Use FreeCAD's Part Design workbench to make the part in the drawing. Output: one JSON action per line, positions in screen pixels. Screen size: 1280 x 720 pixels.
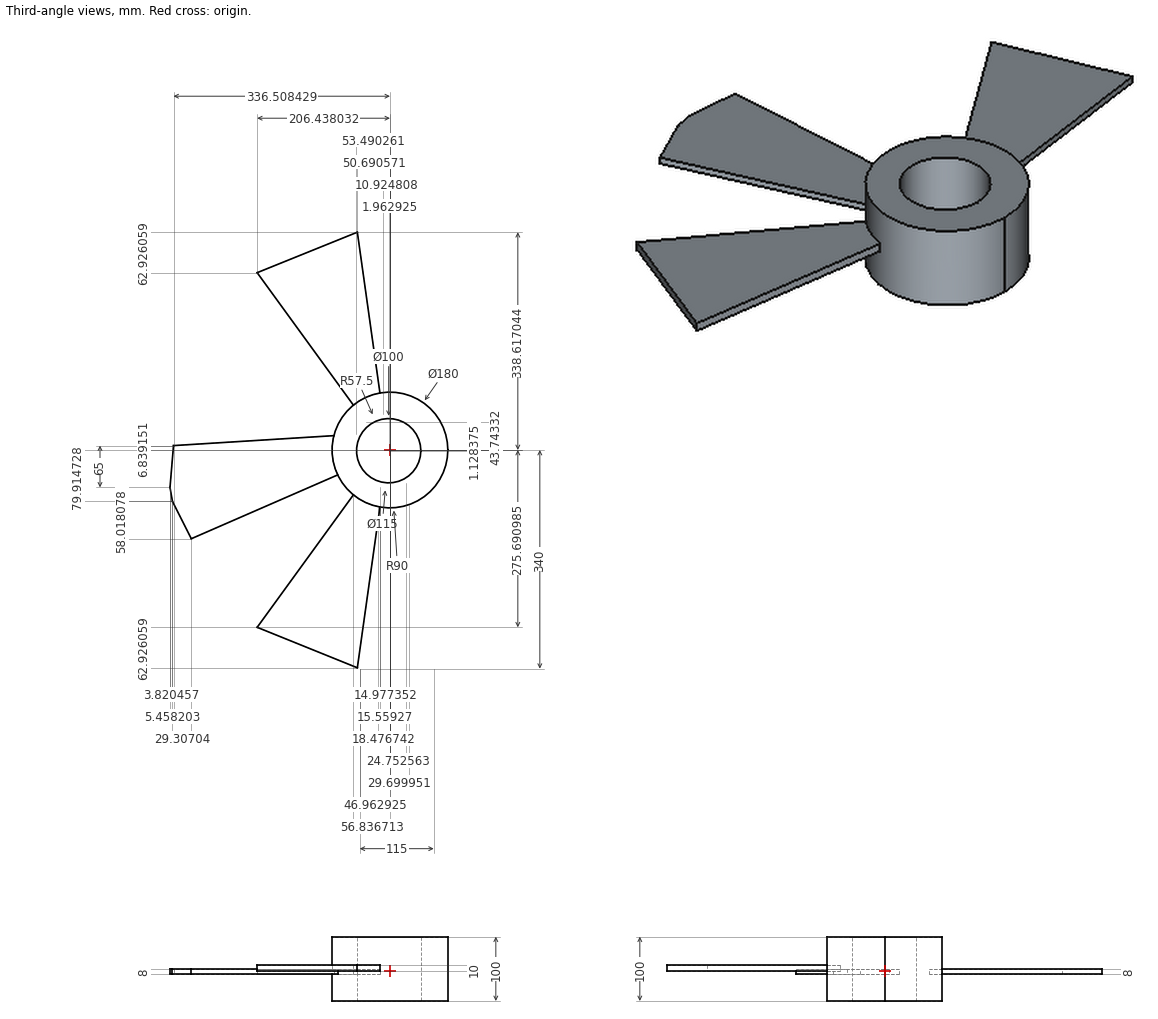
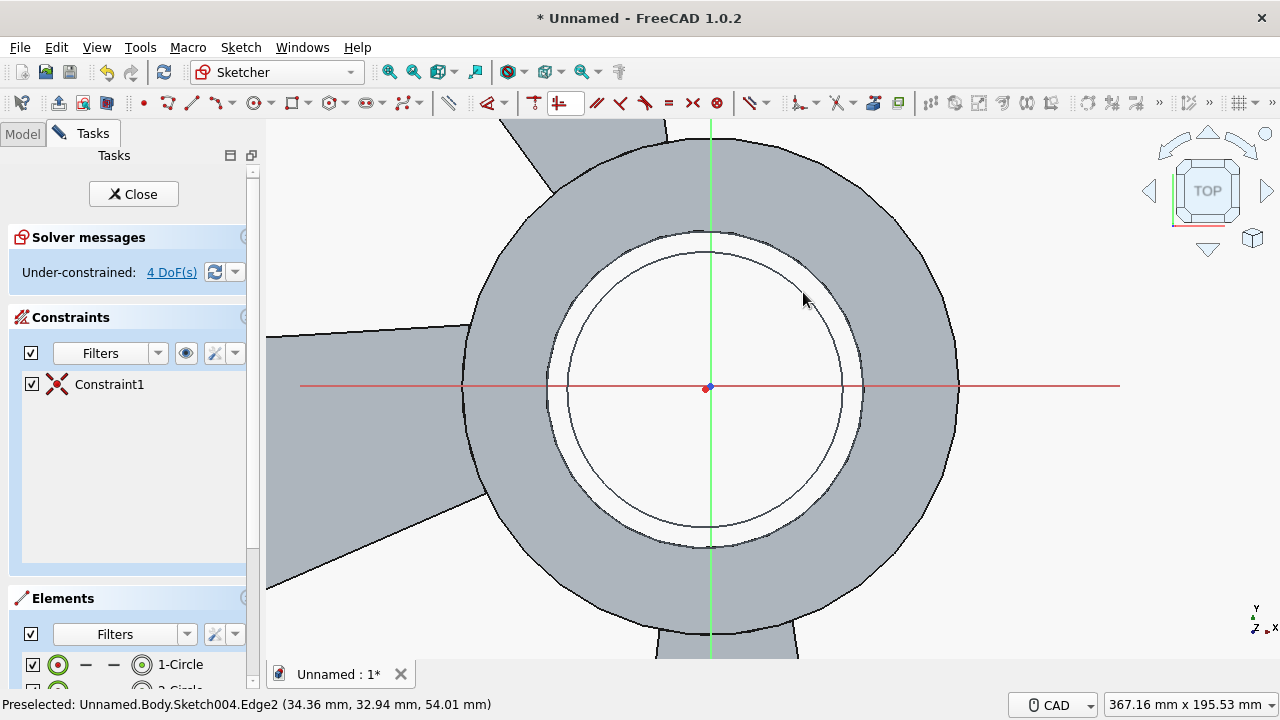
{"action": "left_click", "coordinate": [488, 104]}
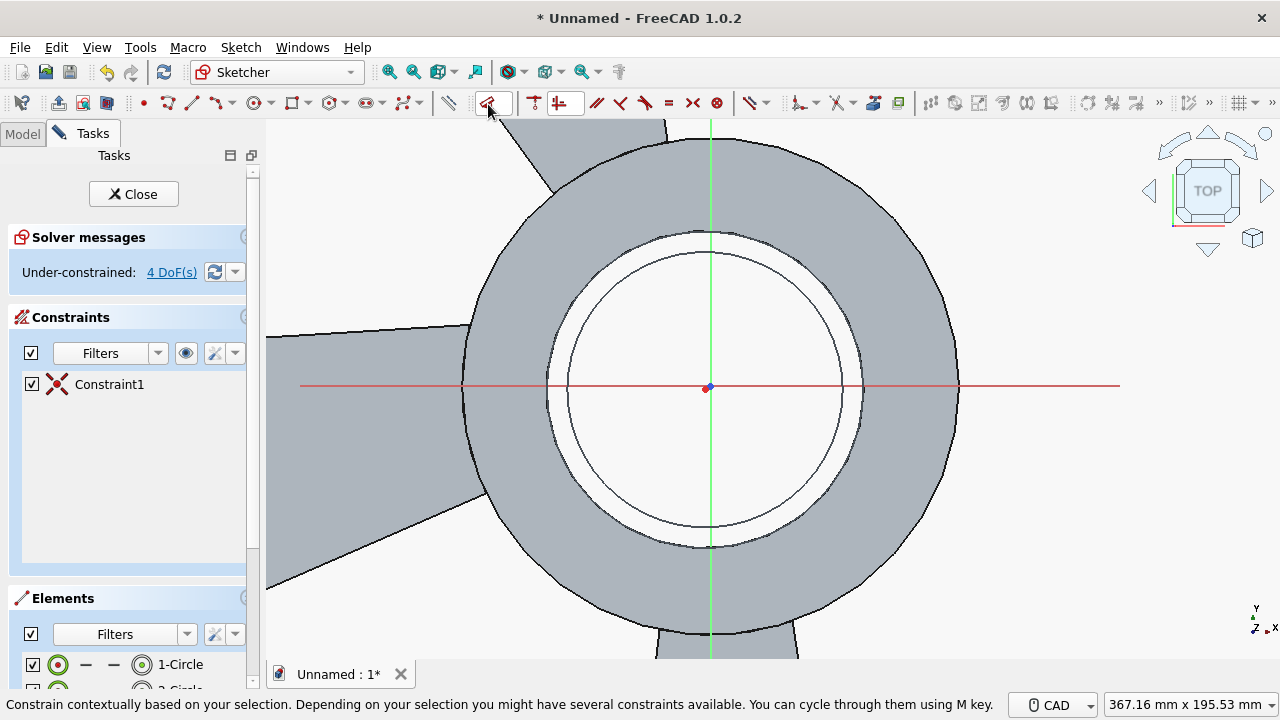
{"action": "left_click", "coordinate": [817, 278]}
{"action": "left_click", "coordinate": [840, 255]}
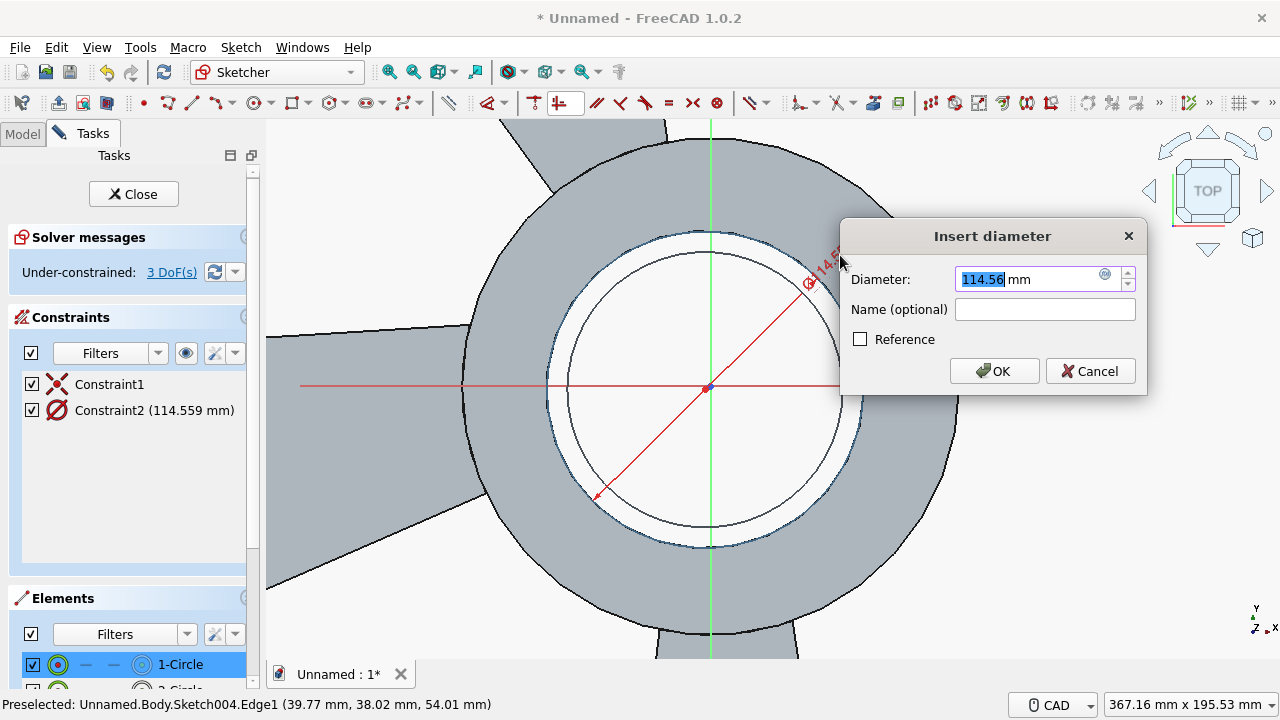
{"action": "type", "text": "115"}
{"action": "key", "text": "Return"}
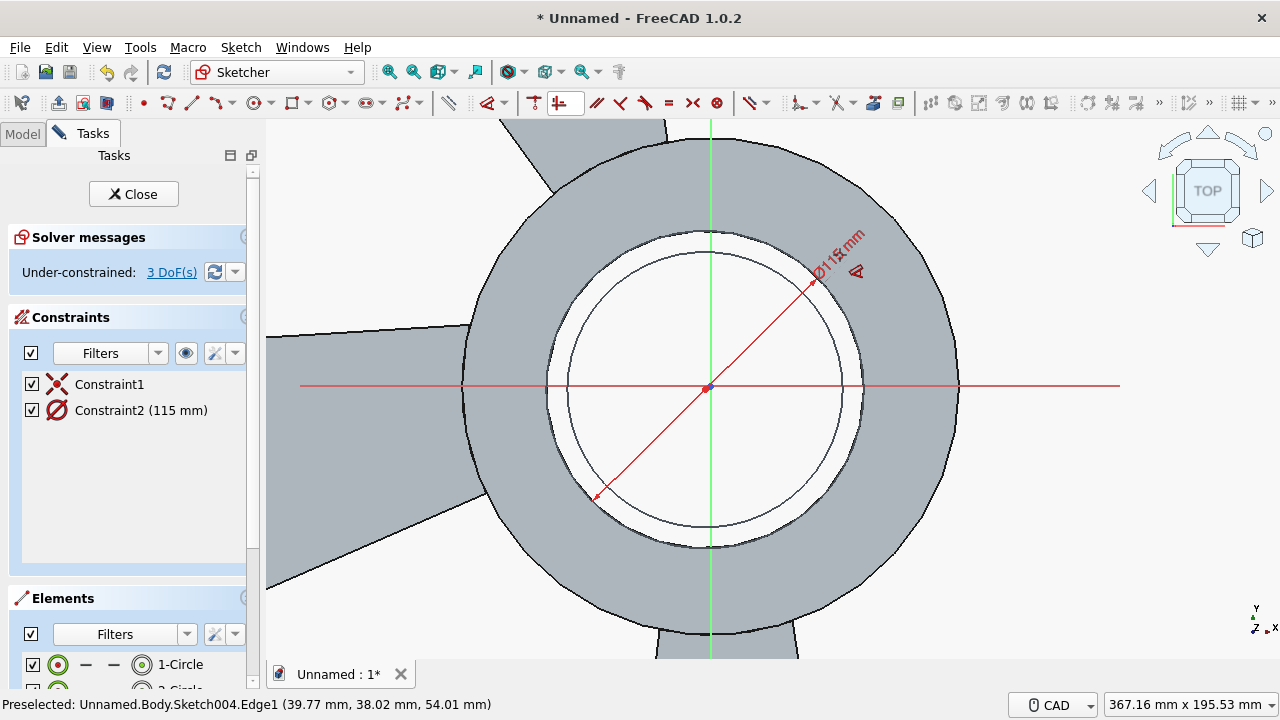
{"action": "left_click", "coordinate": [802, 292]}
{"action": "left_click", "coordinate": [890, 335]}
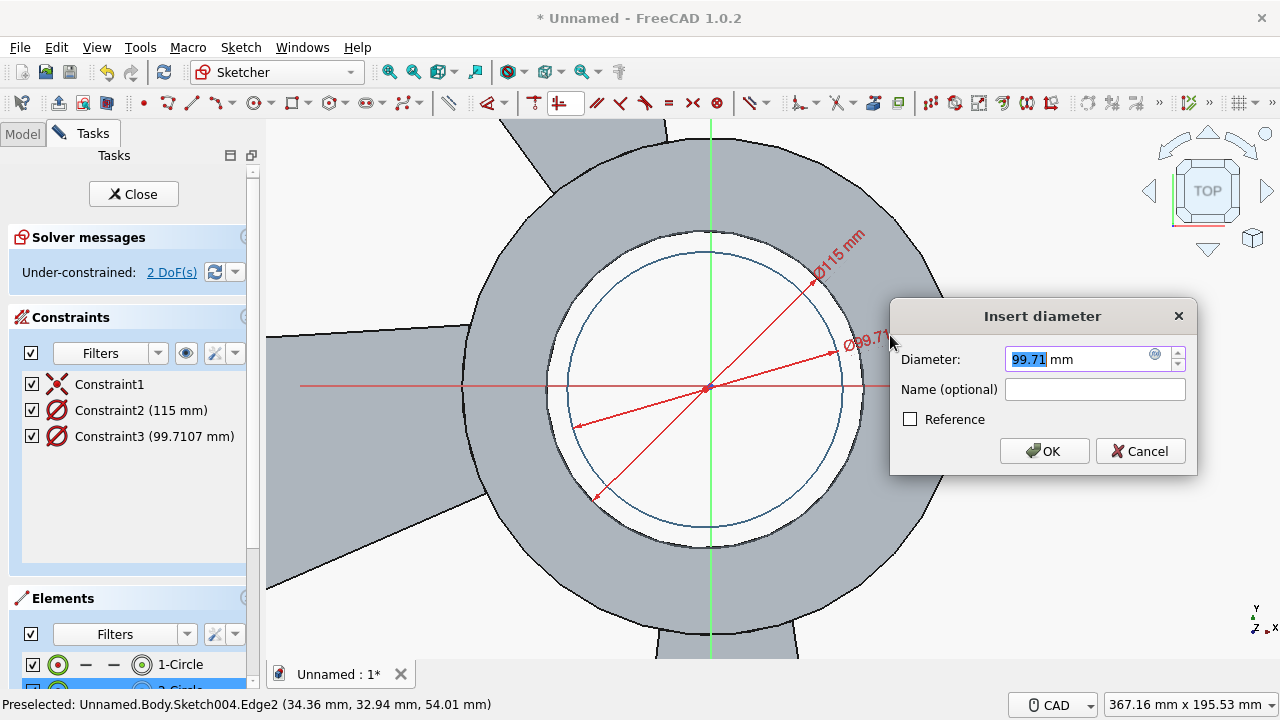
{"action": "type", "text": "100"}
{"action": "key", "text": "Return"}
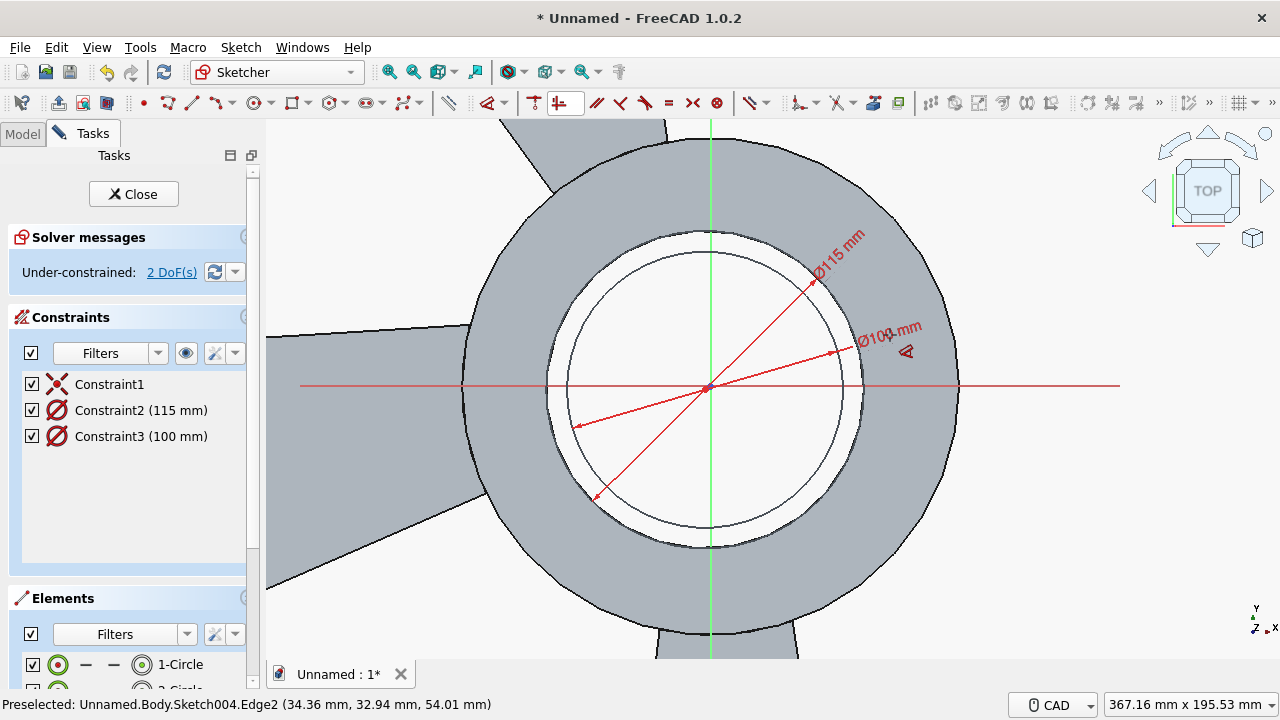
{"action": "scroll", "coordinate": [705, 390], "scroll_direction": "up", "scroll_amount": 10}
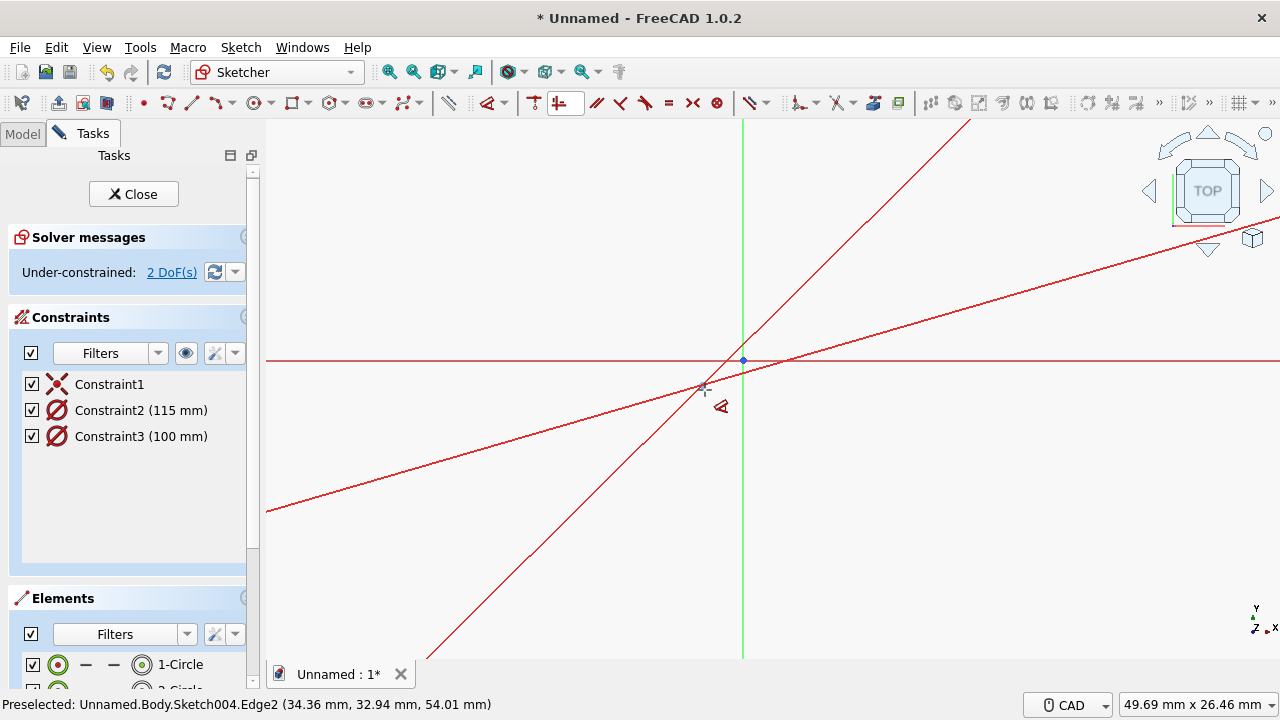
{"action": "left_click", "coordinate": [703, 385]}
{"action": "left_click", "coordinate": [723, 327]}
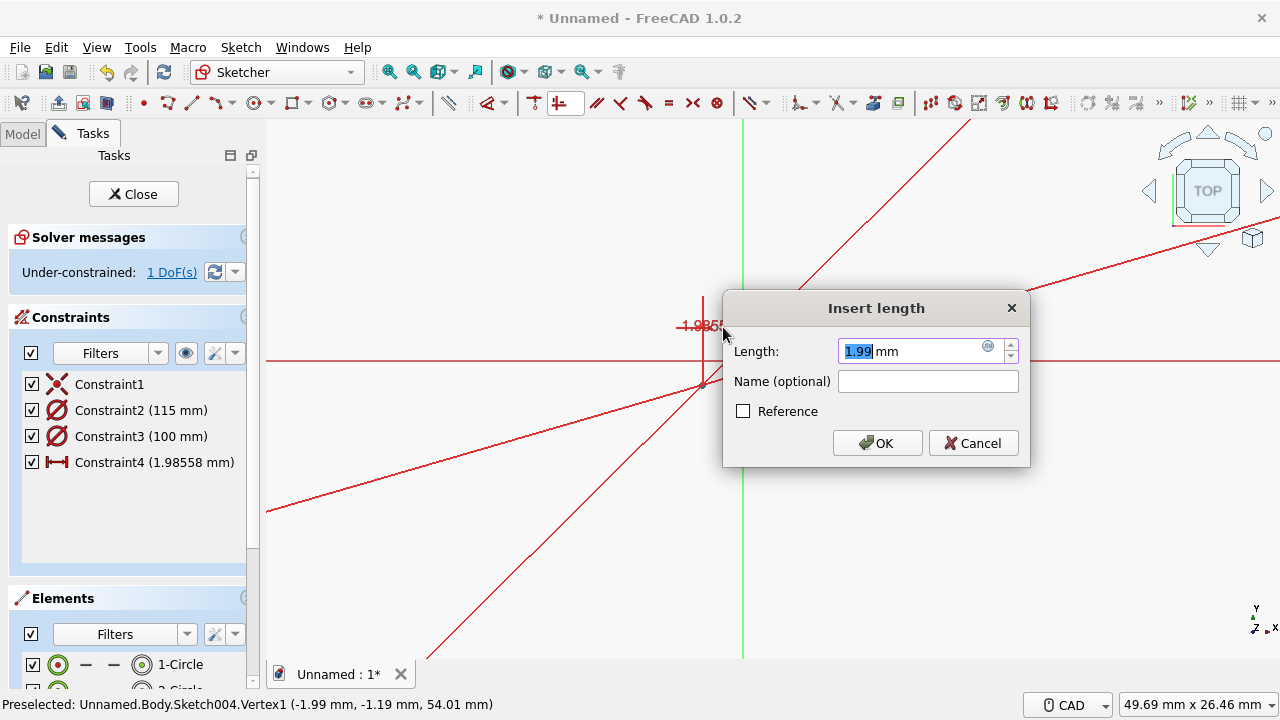
{"action": "type", "text": "1.962925"}
{"action": "key", "text": "Return"}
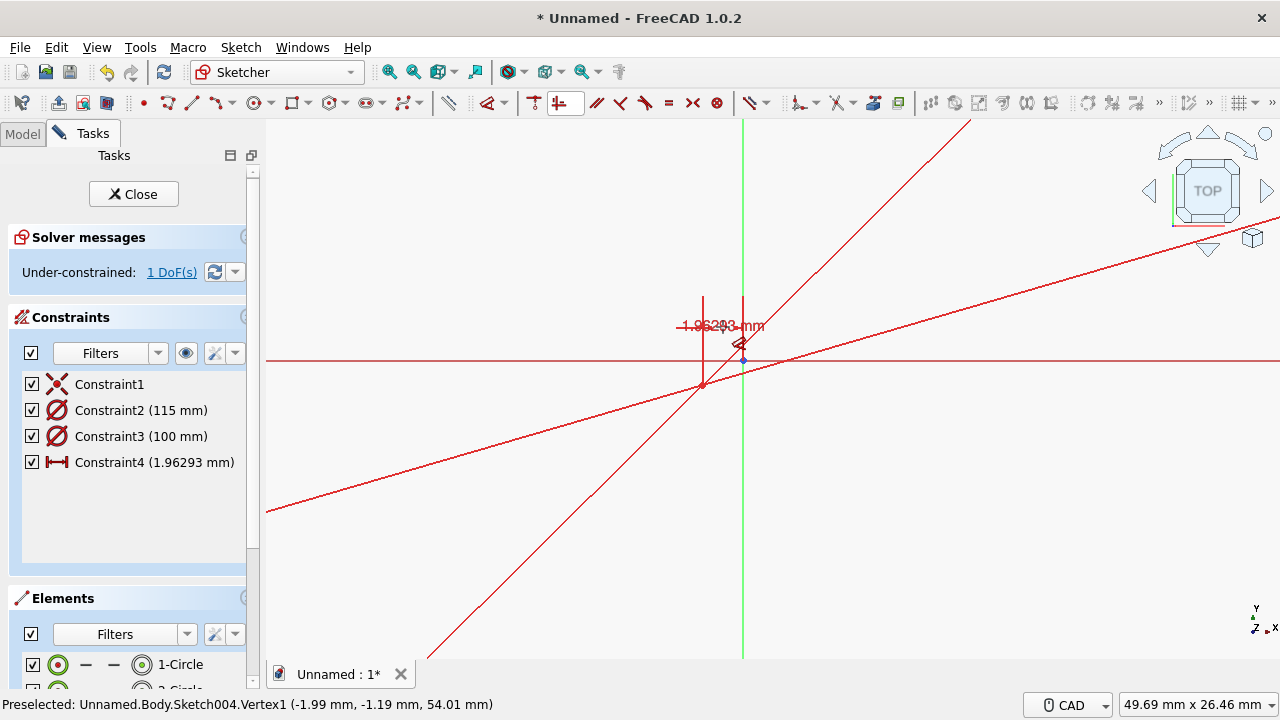
{"action": "scroll", "coordinate": [703, 385], "scroll_direction": "up", "scroll_amount": 3}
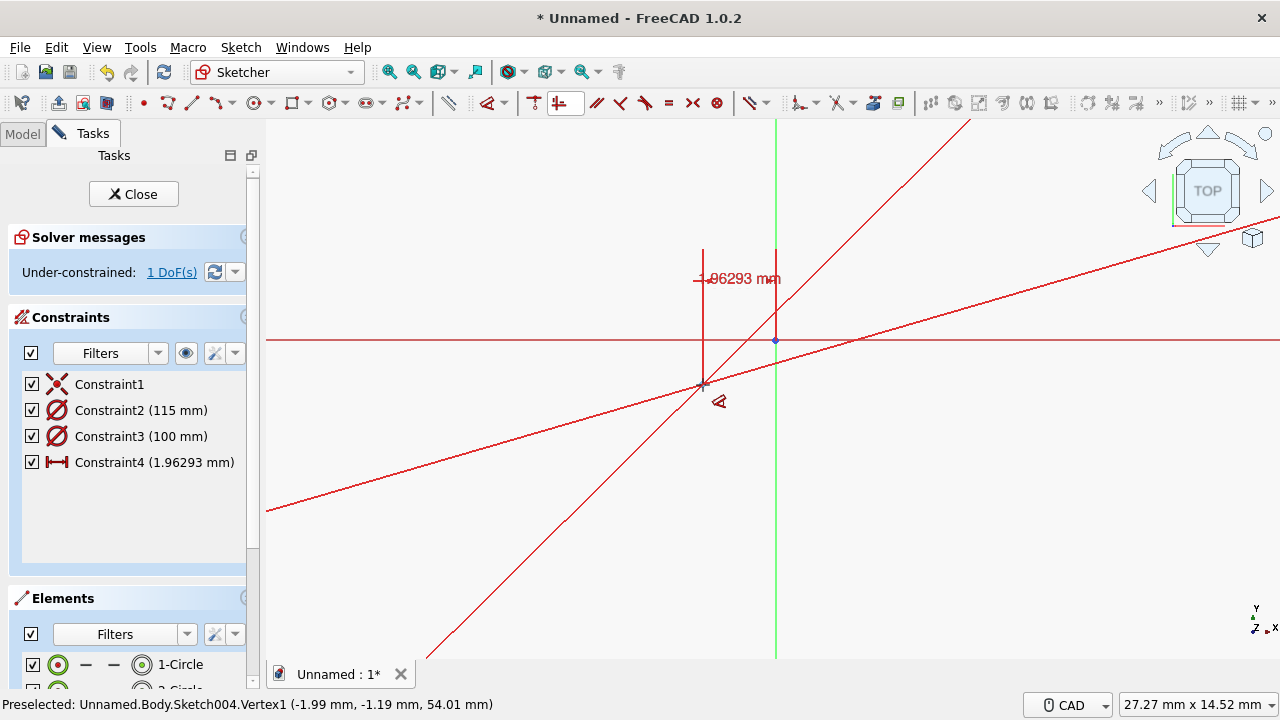
{"action": "left_click", "coordinate": [703, 385]}
{"action": "left_click", "coordinate": [810, 362]}